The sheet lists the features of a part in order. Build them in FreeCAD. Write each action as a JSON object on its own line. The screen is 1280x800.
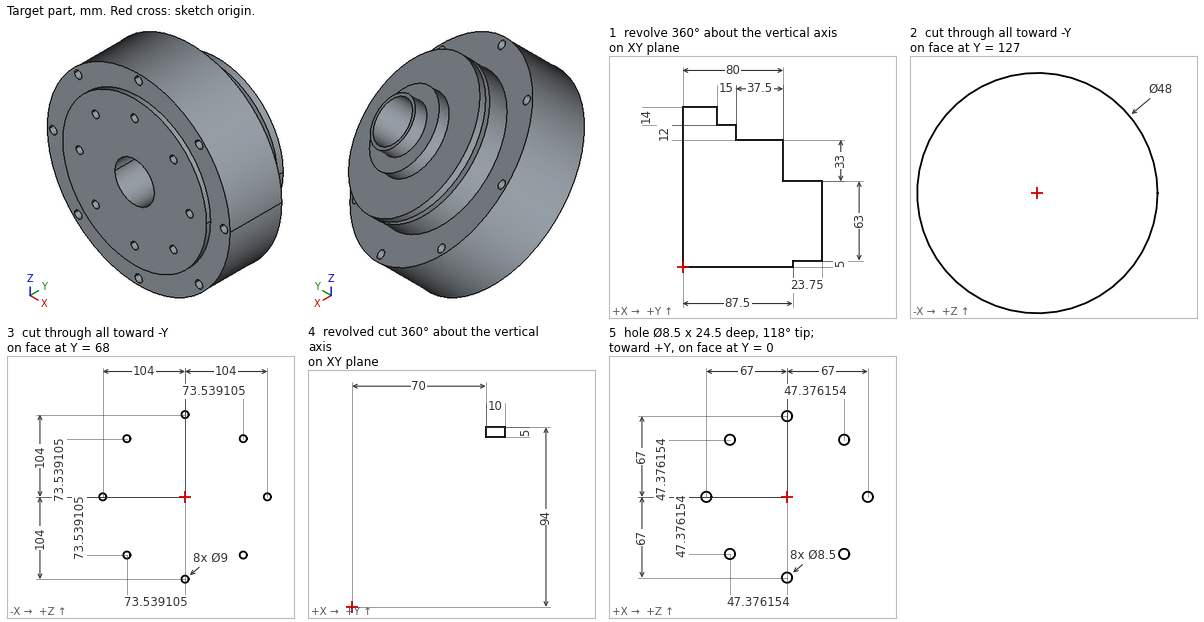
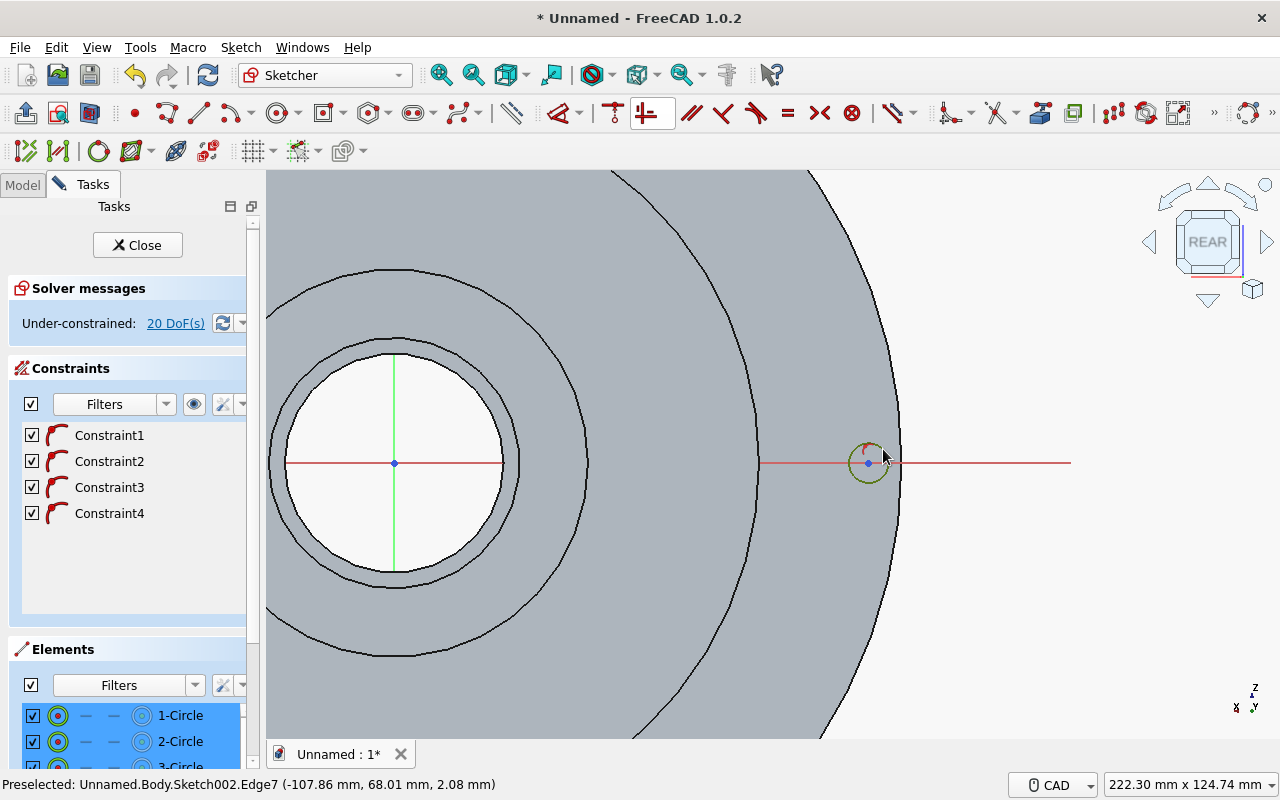
{"action": "scroll", "coordinate": [885, 449], "scroll_direction": "down", "scroll_amount": 5}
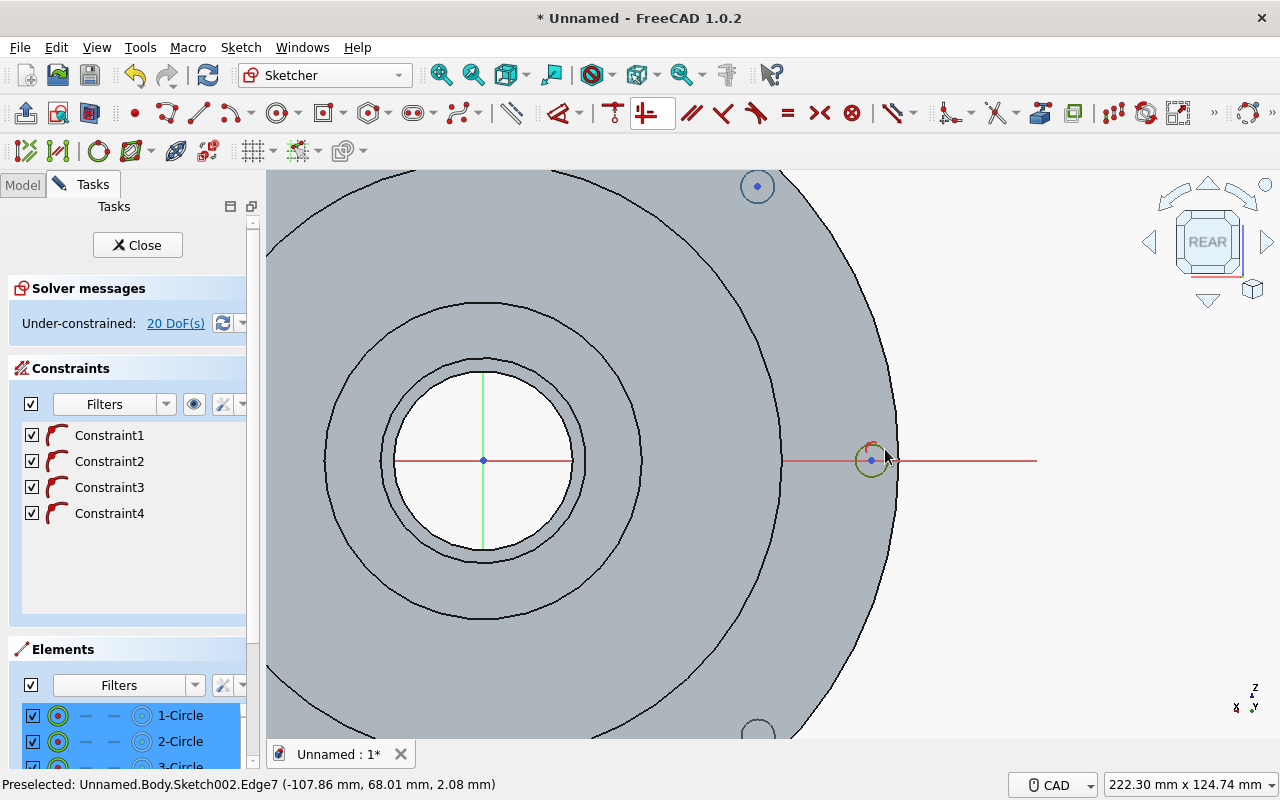
{"action": "scroll", "coordinate": [834, 573], "scroll_direction": "up", "scroll_amount": 4}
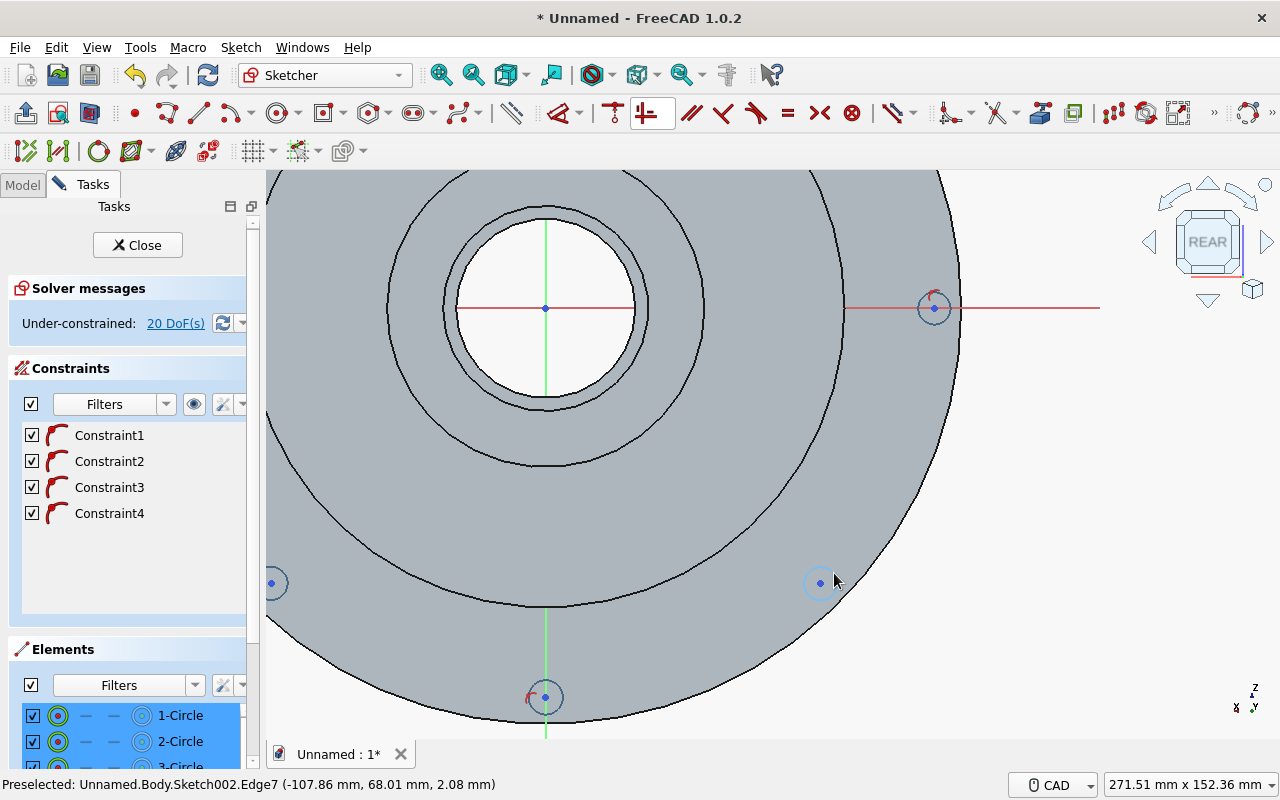
{"action": "left_click", "coordinate": [832, 572]}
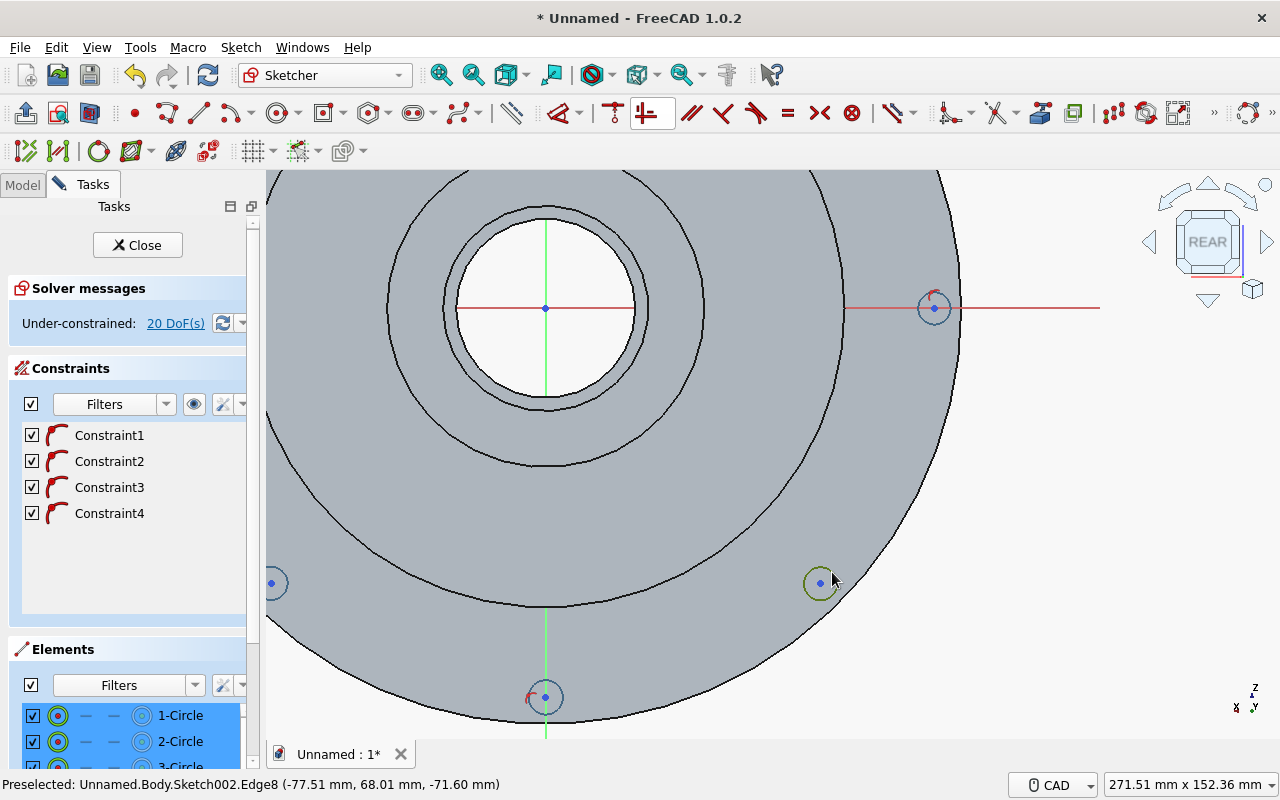
{"action": "left_click", "coordinate": [788, 114]}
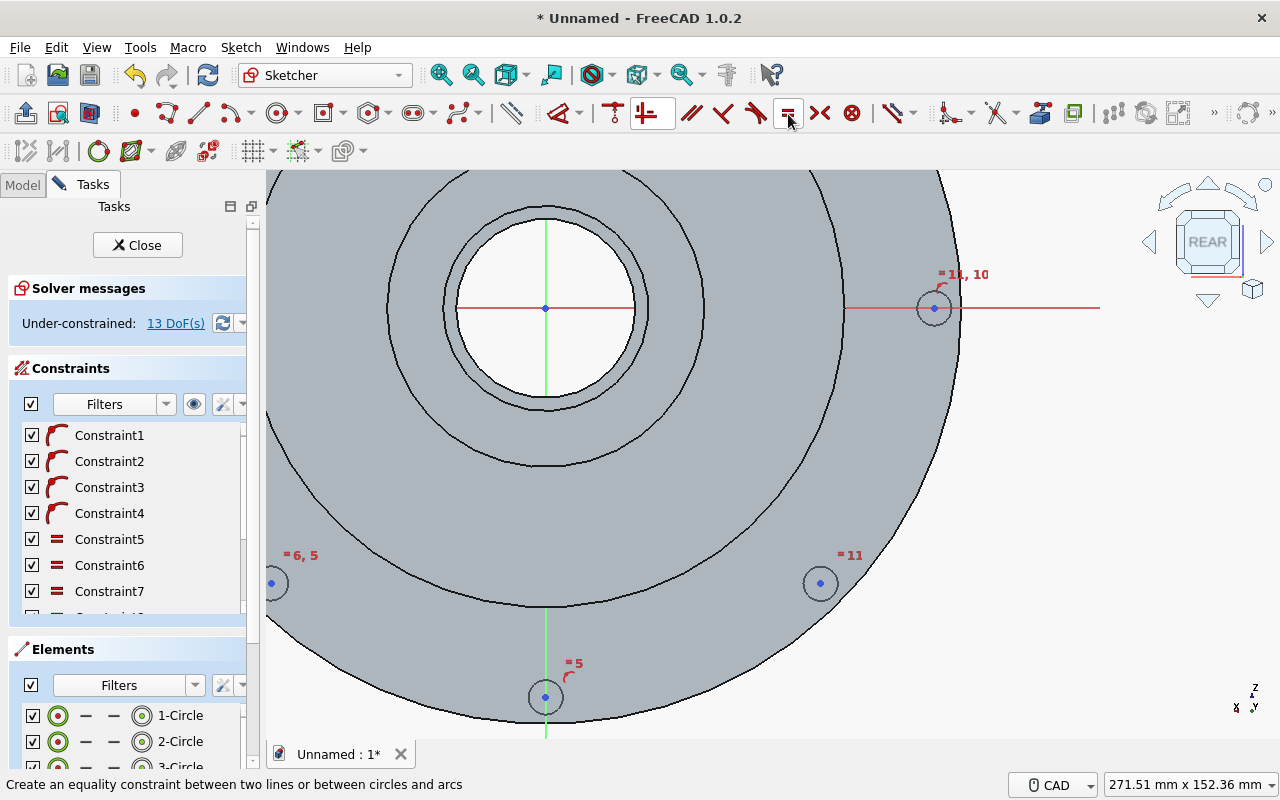
{"action": "scroll", "coordinate": [834, 574], "scroll_direction": "down", "scroll_amount": 4}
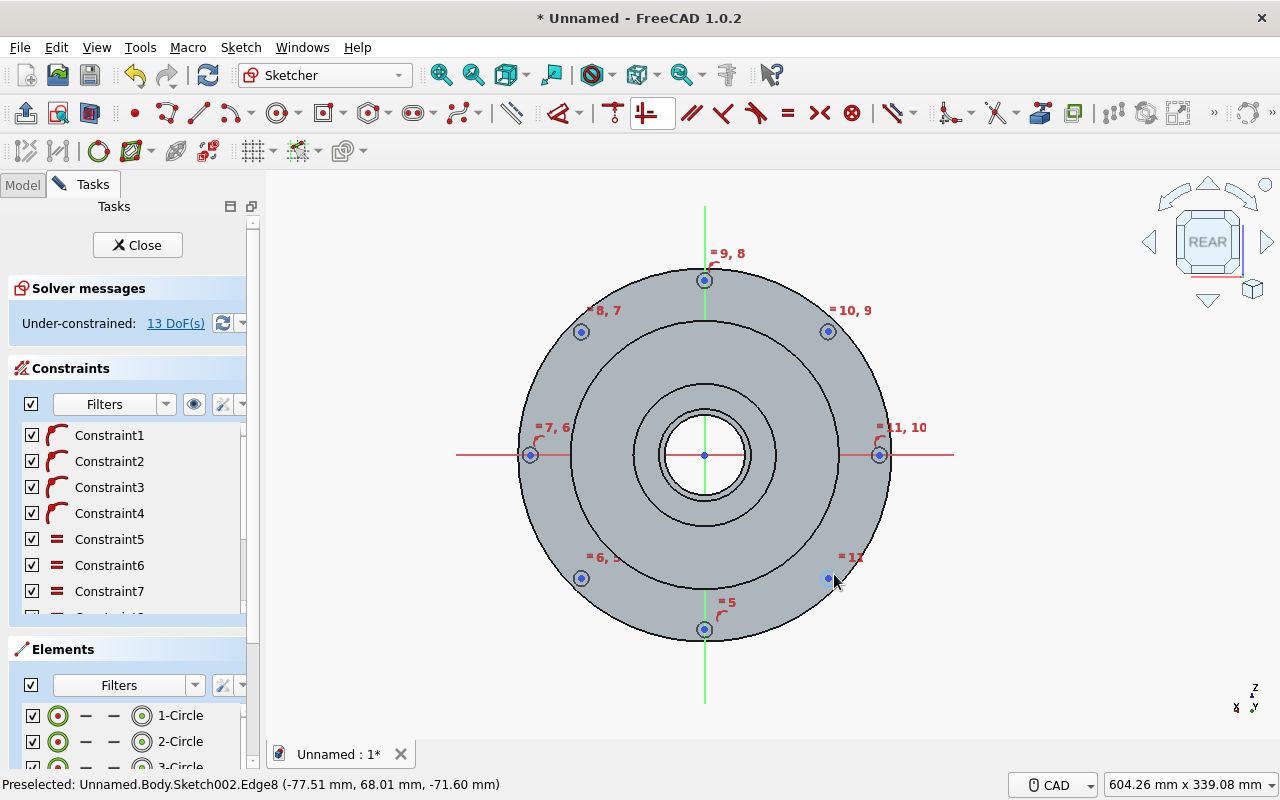
{"action": "left_click", "coordinate": [581, 579]}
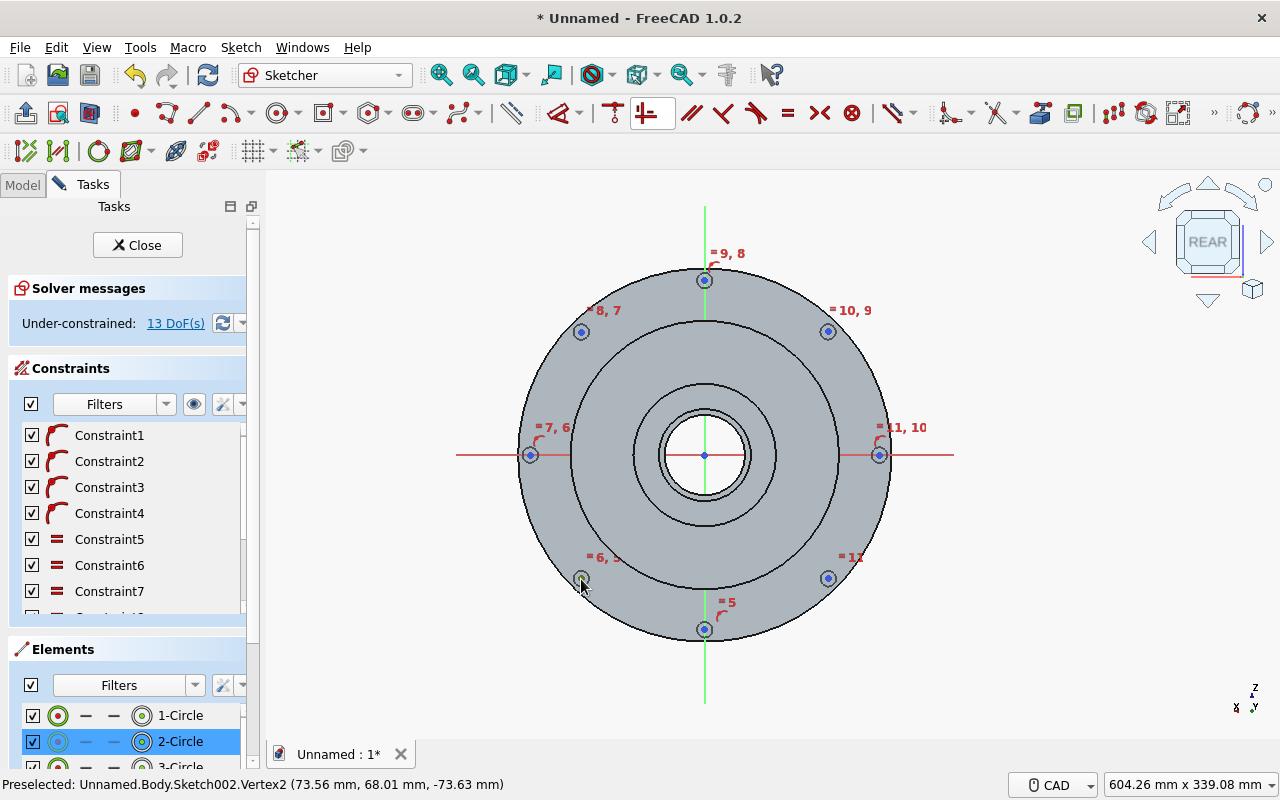
{"action": "left_click", "coordinate": [581, 332]}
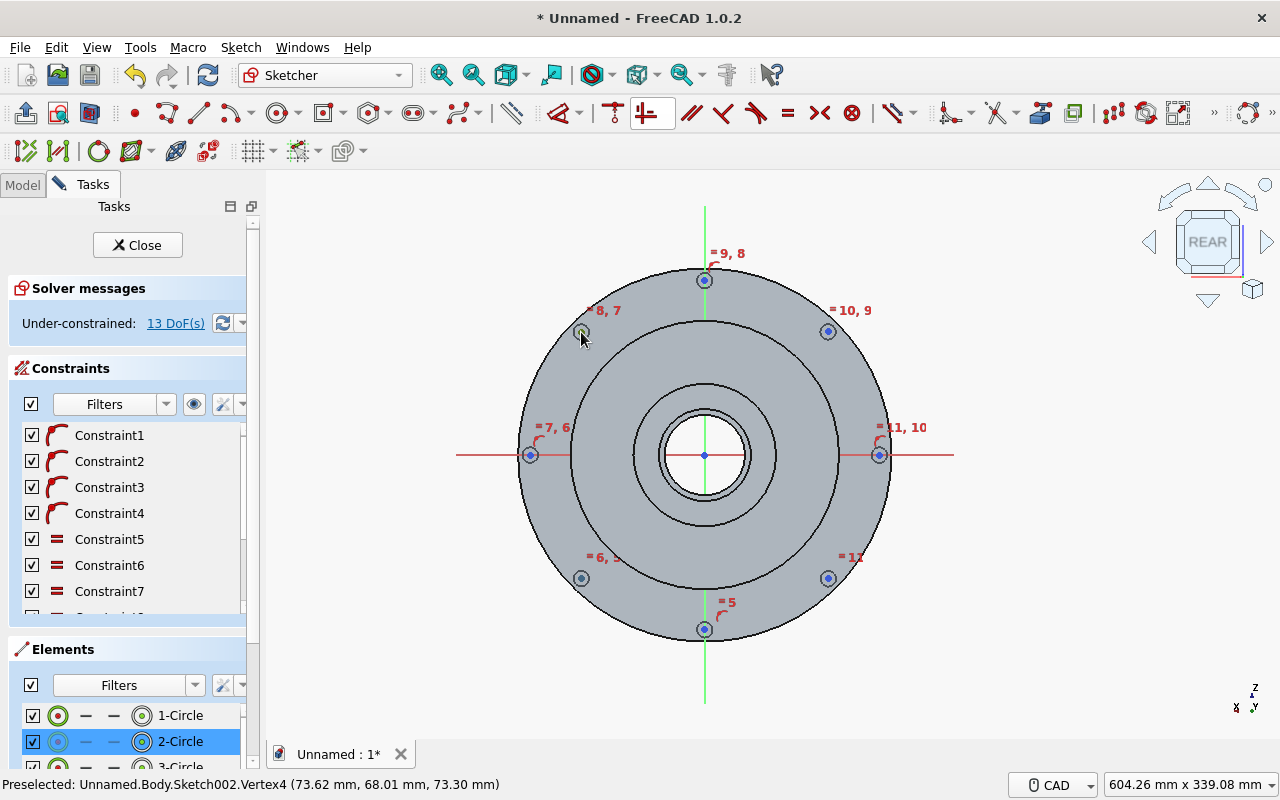
{"action": "left_click", "coordinate": [670, 114]}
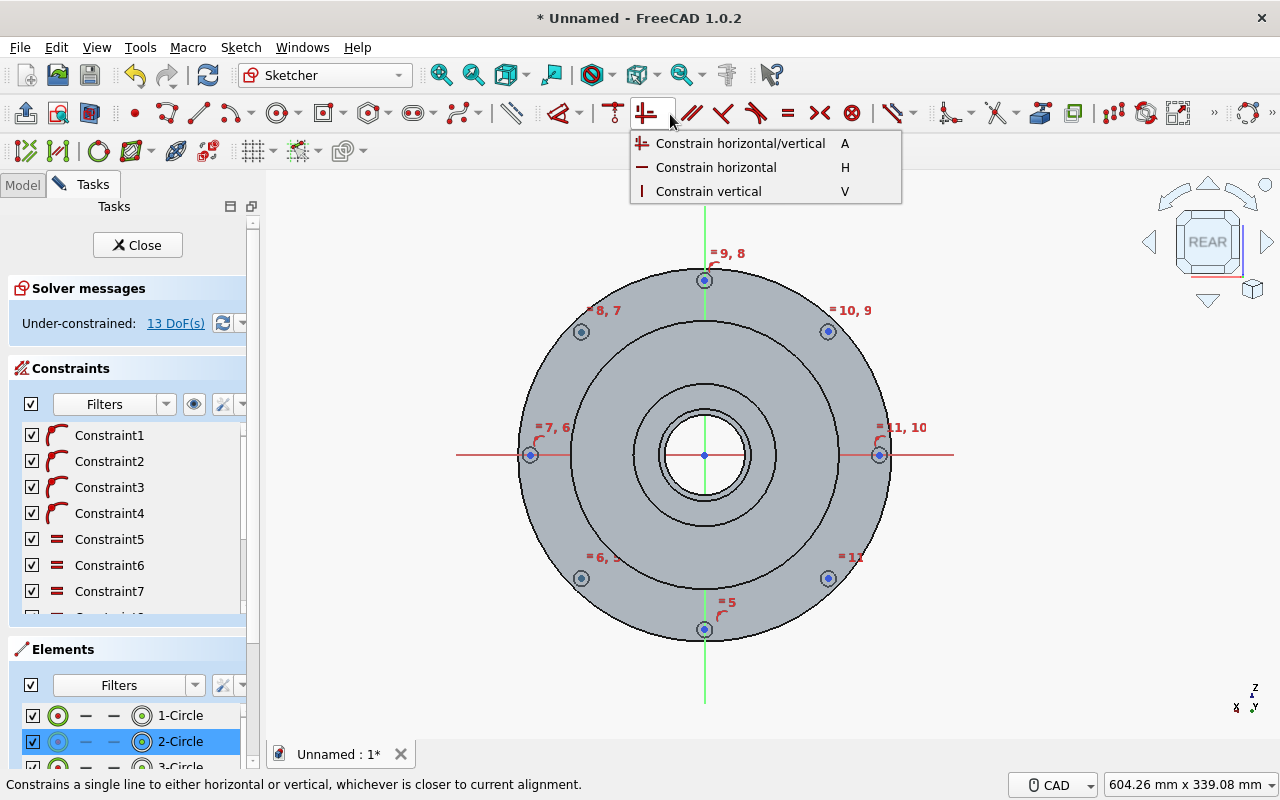
{"action": "left_click", "coordinate": [766, 191]}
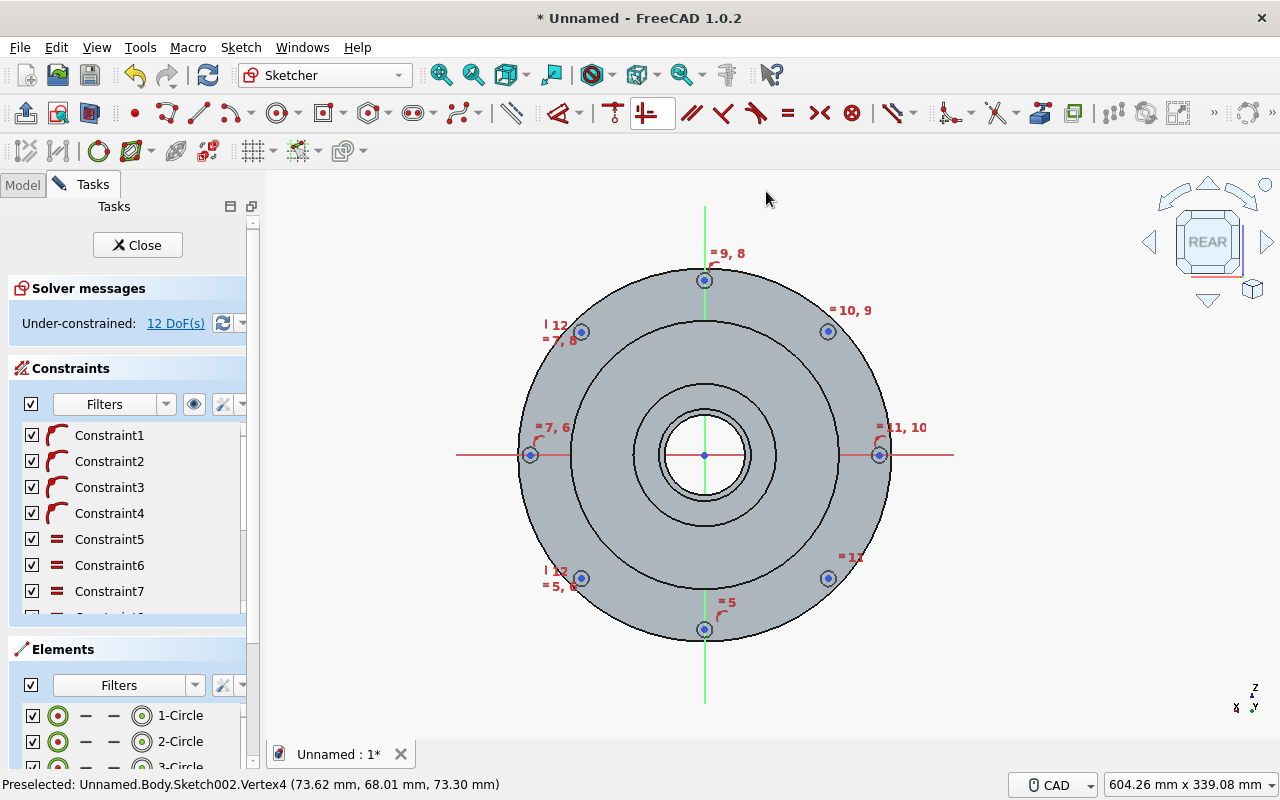
{"action": "left_click", "coordinate": [581, 332]}